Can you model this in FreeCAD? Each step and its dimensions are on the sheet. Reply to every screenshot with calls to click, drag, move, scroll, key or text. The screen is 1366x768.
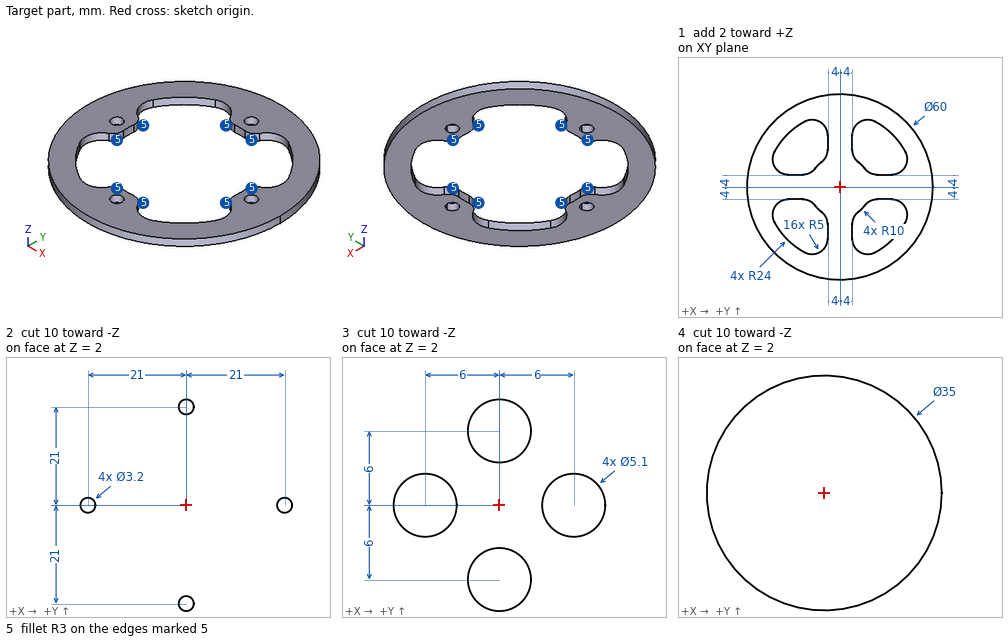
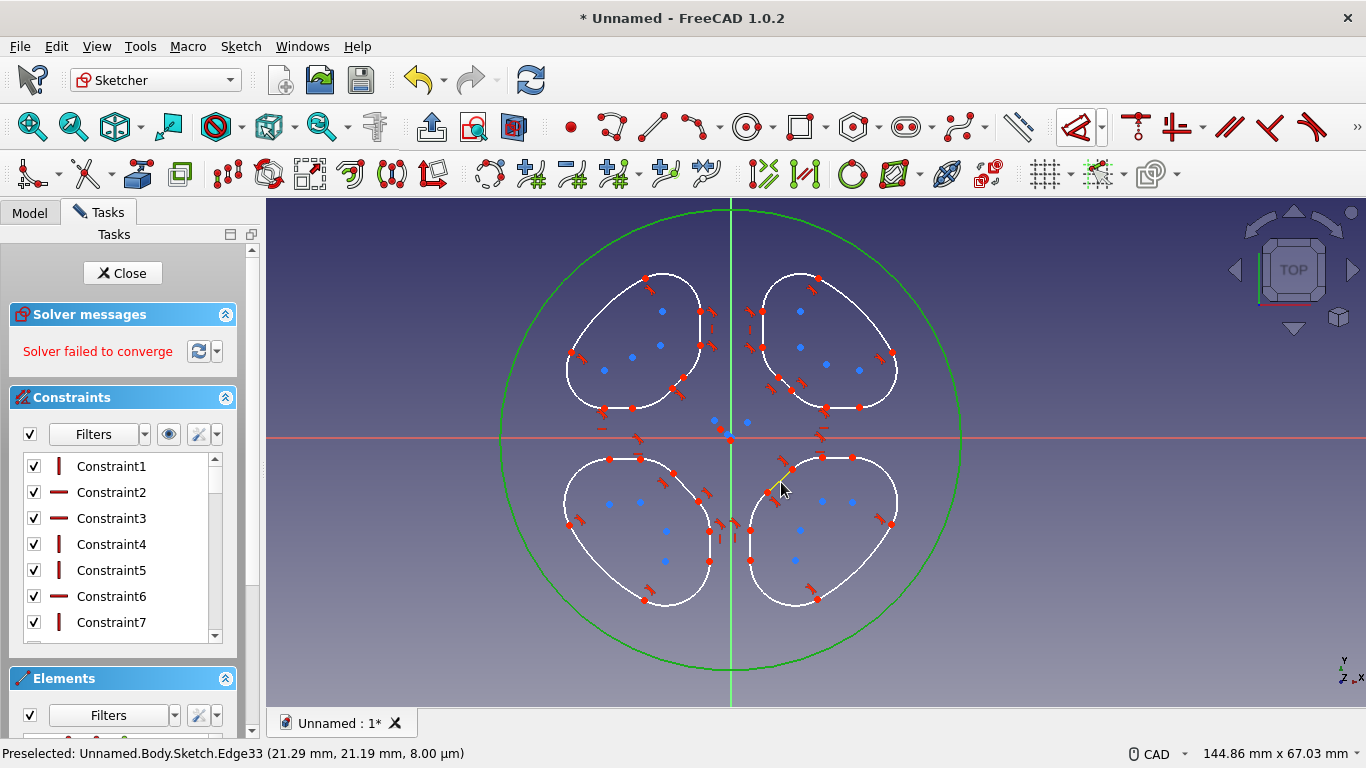
click(780, 481)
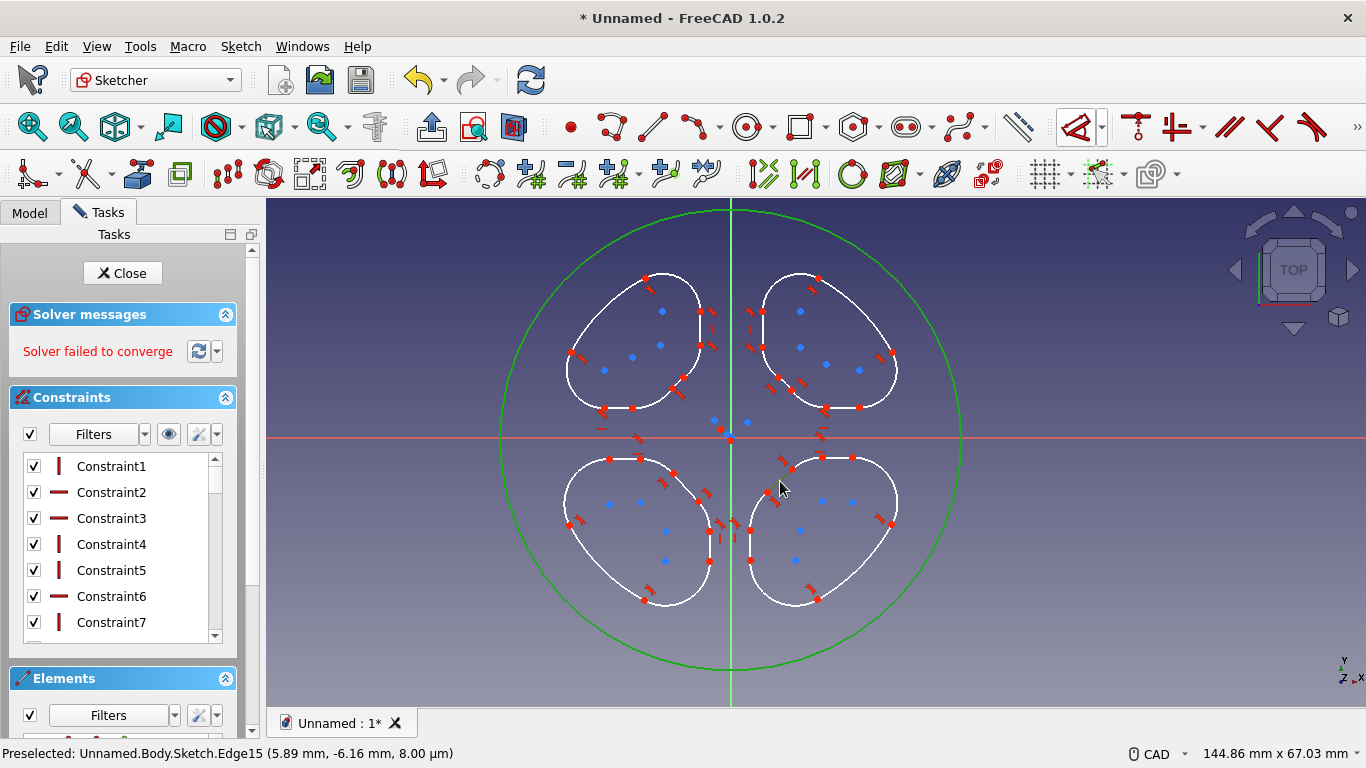
click(1136, 128)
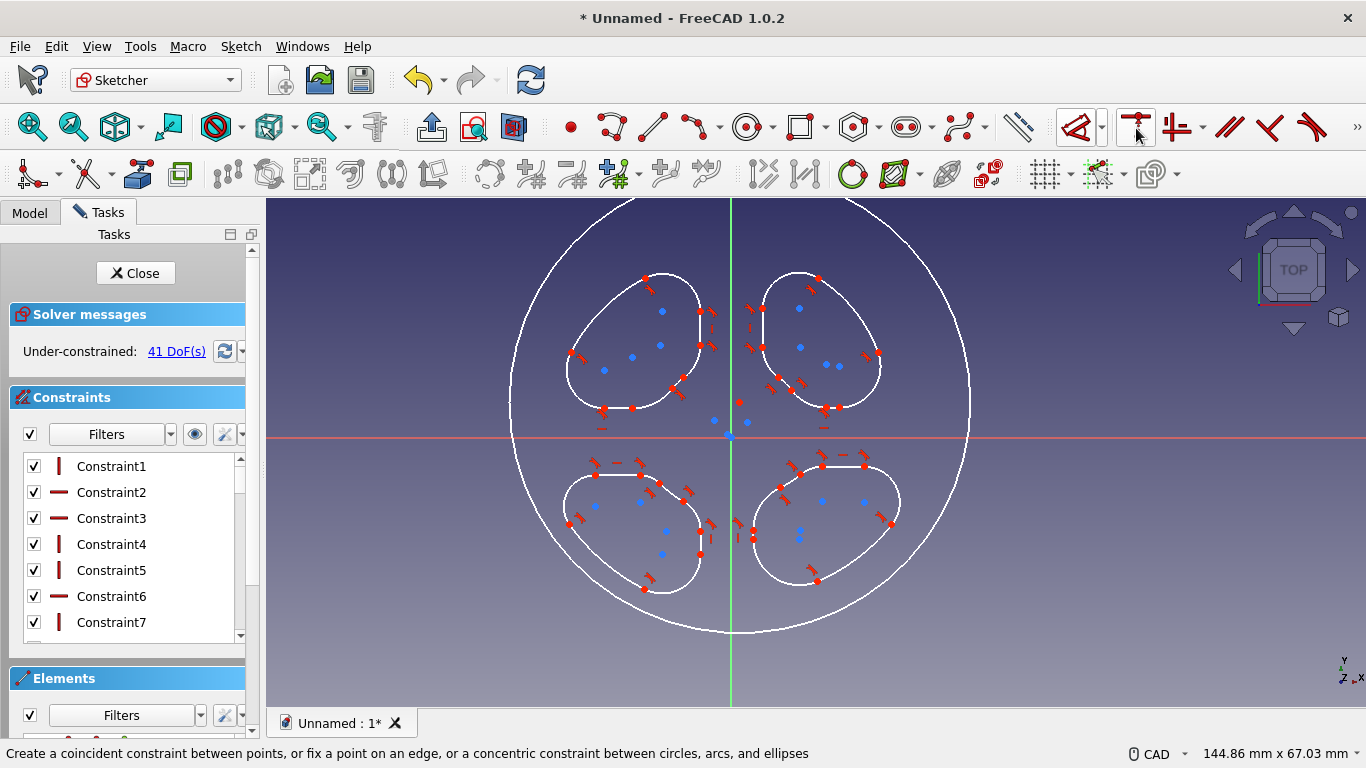
click(902, 239)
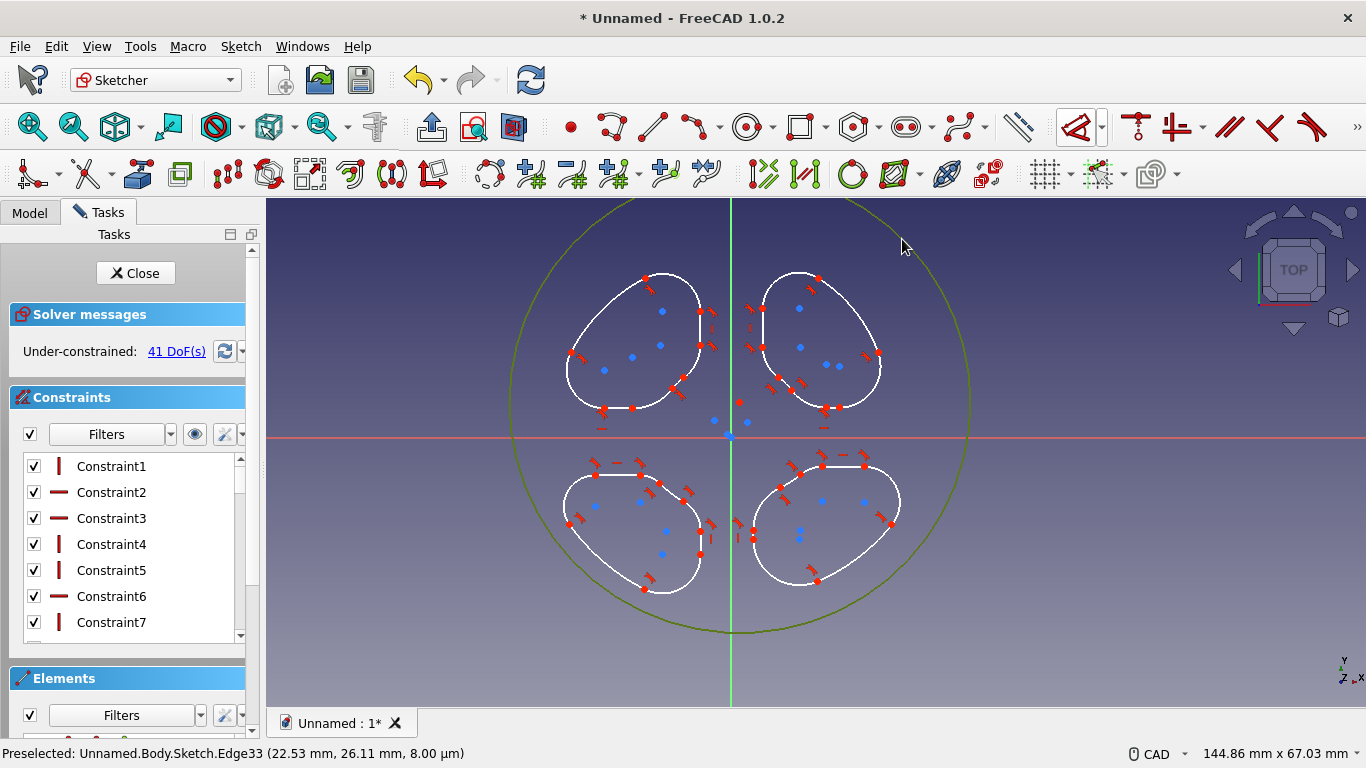
scroll(678, 383, up, 3)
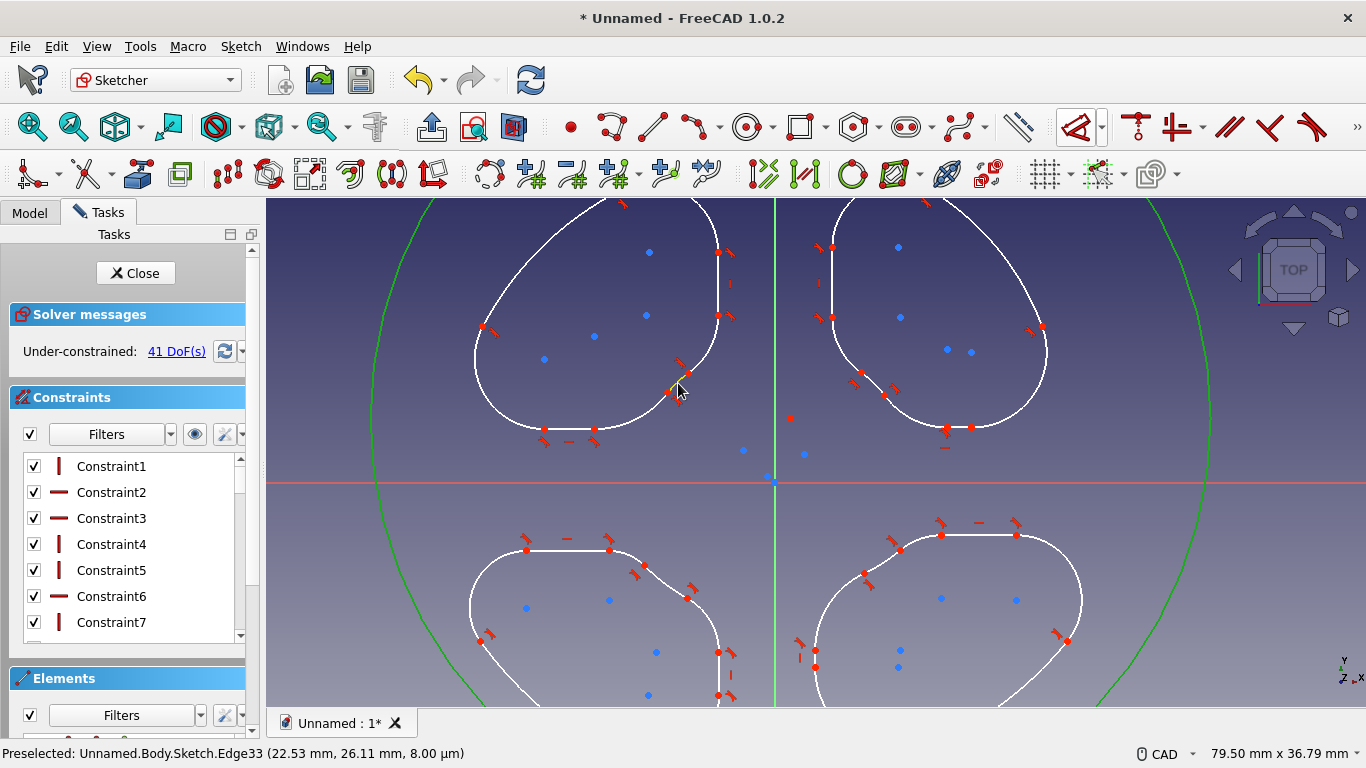
click(677, 382)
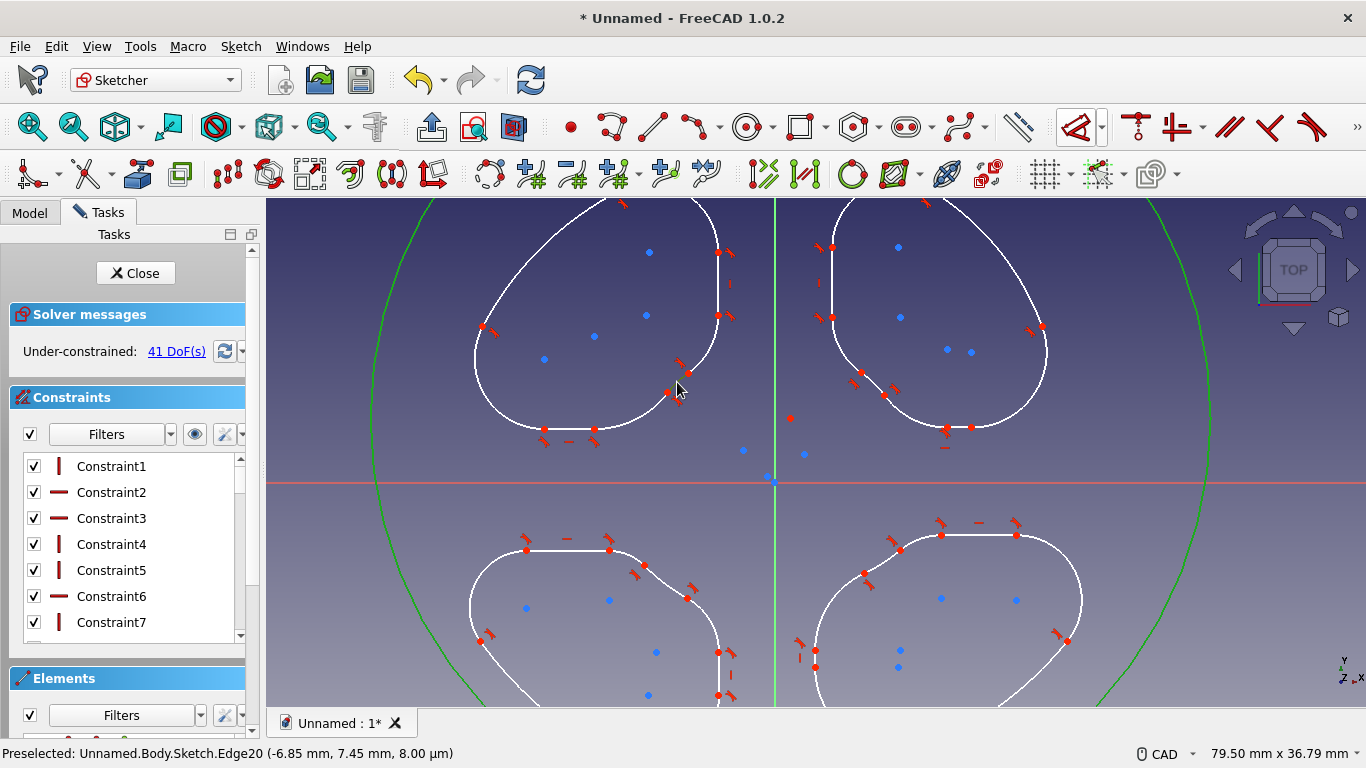
click(1136, 128)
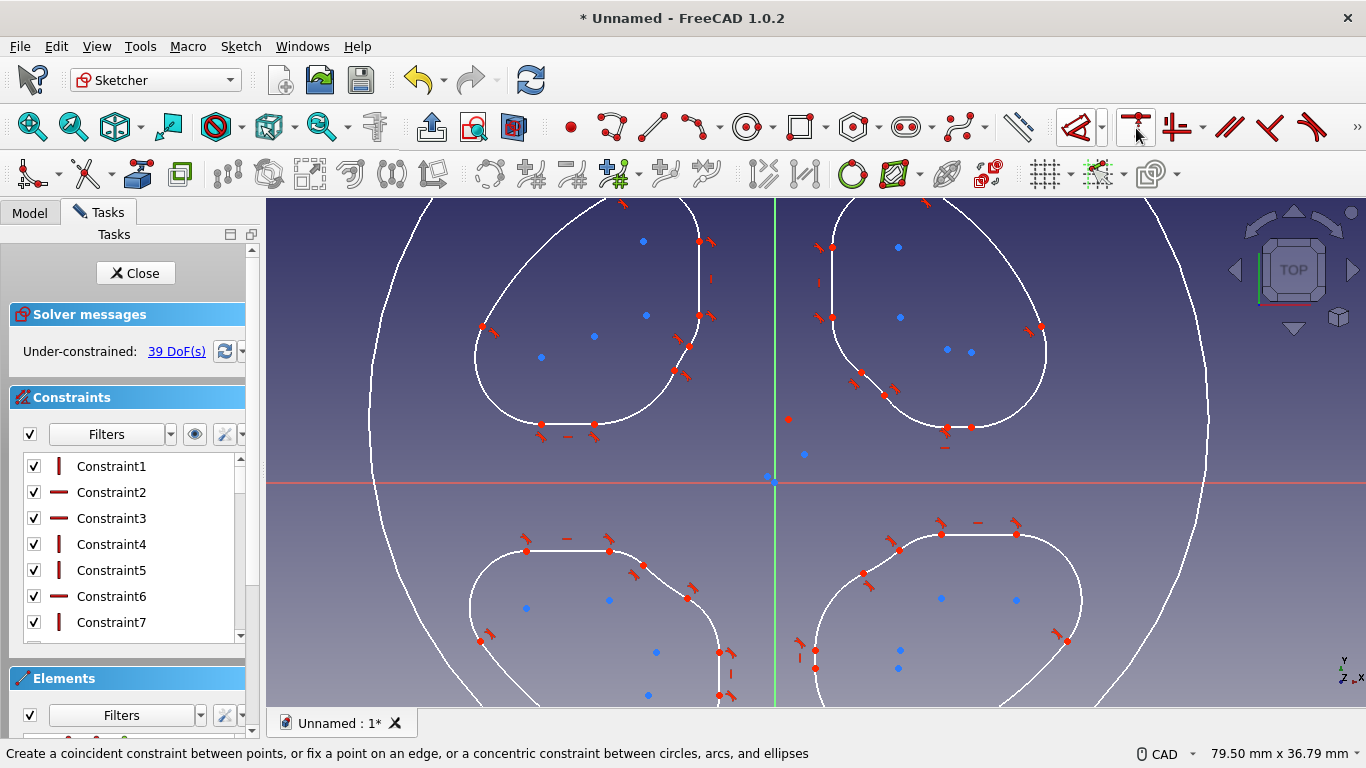
click(369, 407)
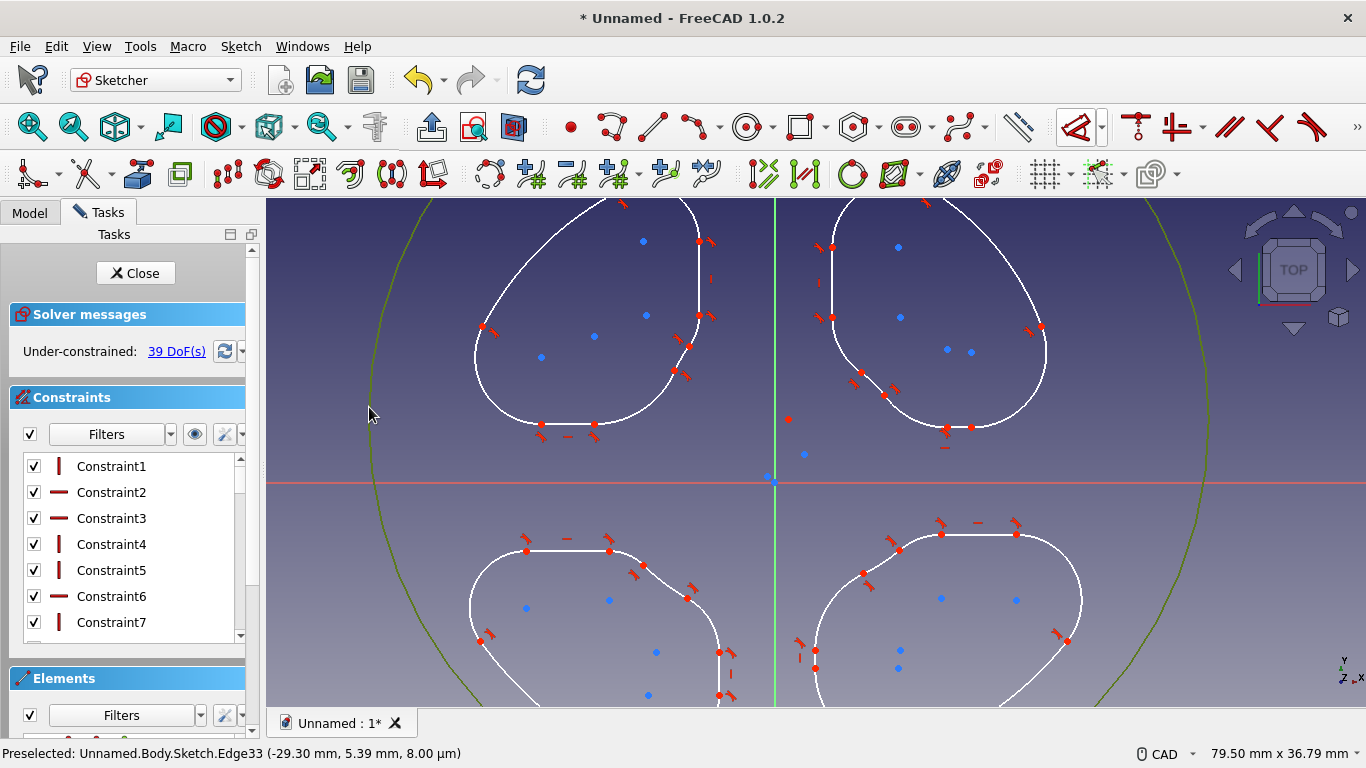
click(514, 278)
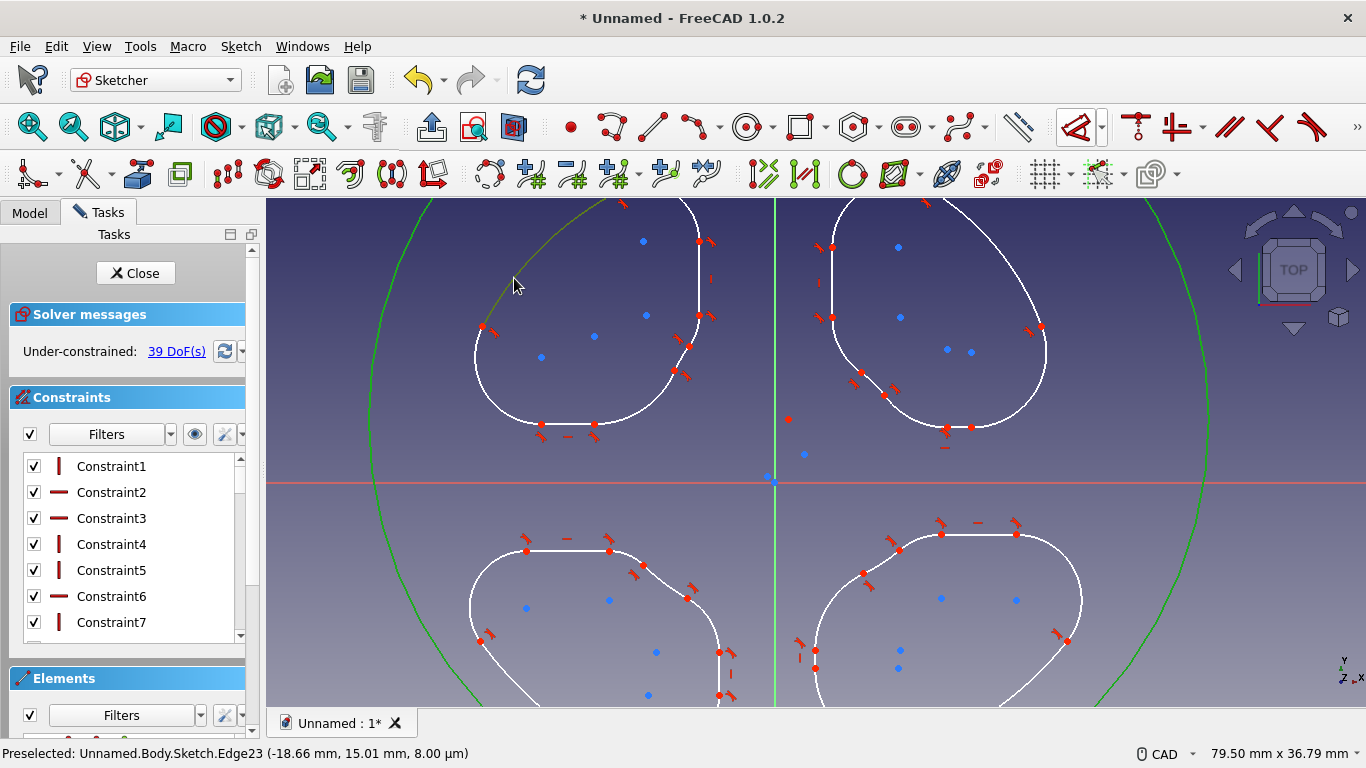
key(c)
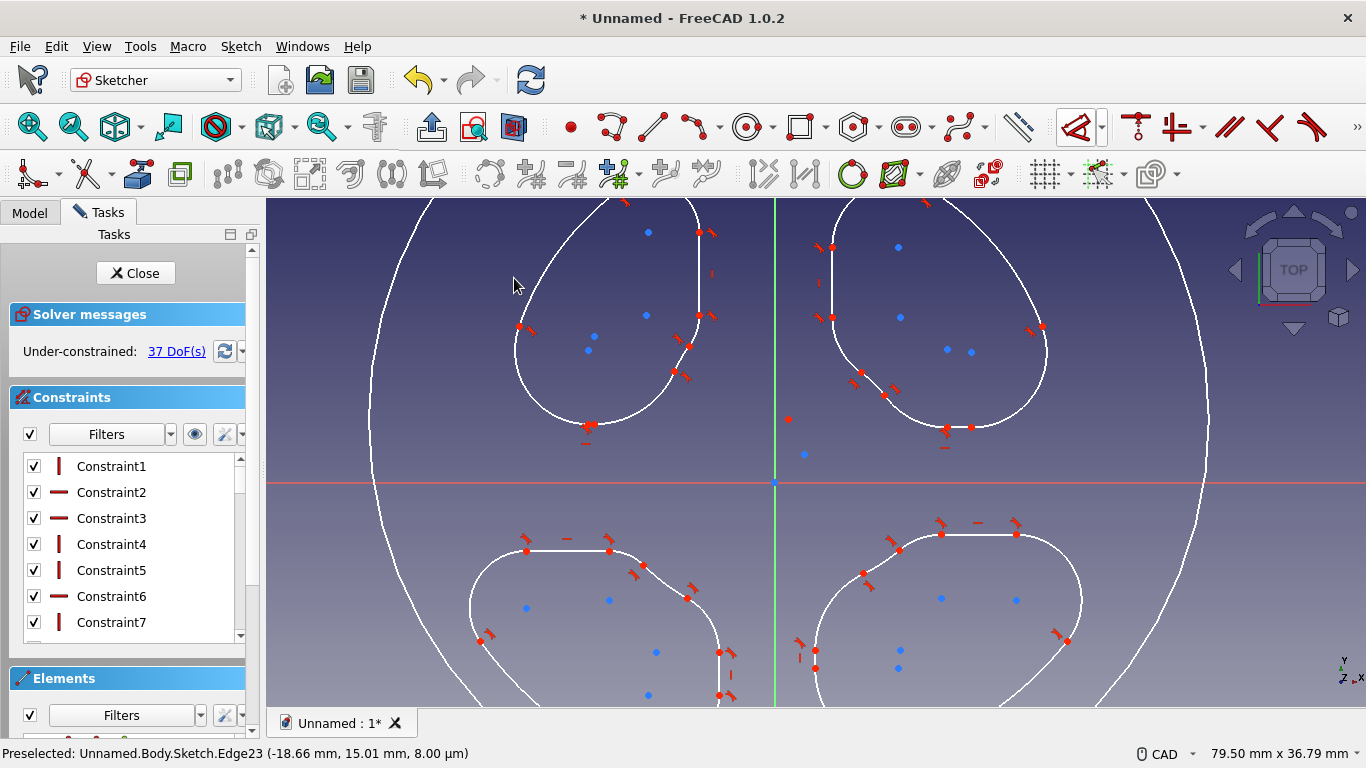
click(369, 408)